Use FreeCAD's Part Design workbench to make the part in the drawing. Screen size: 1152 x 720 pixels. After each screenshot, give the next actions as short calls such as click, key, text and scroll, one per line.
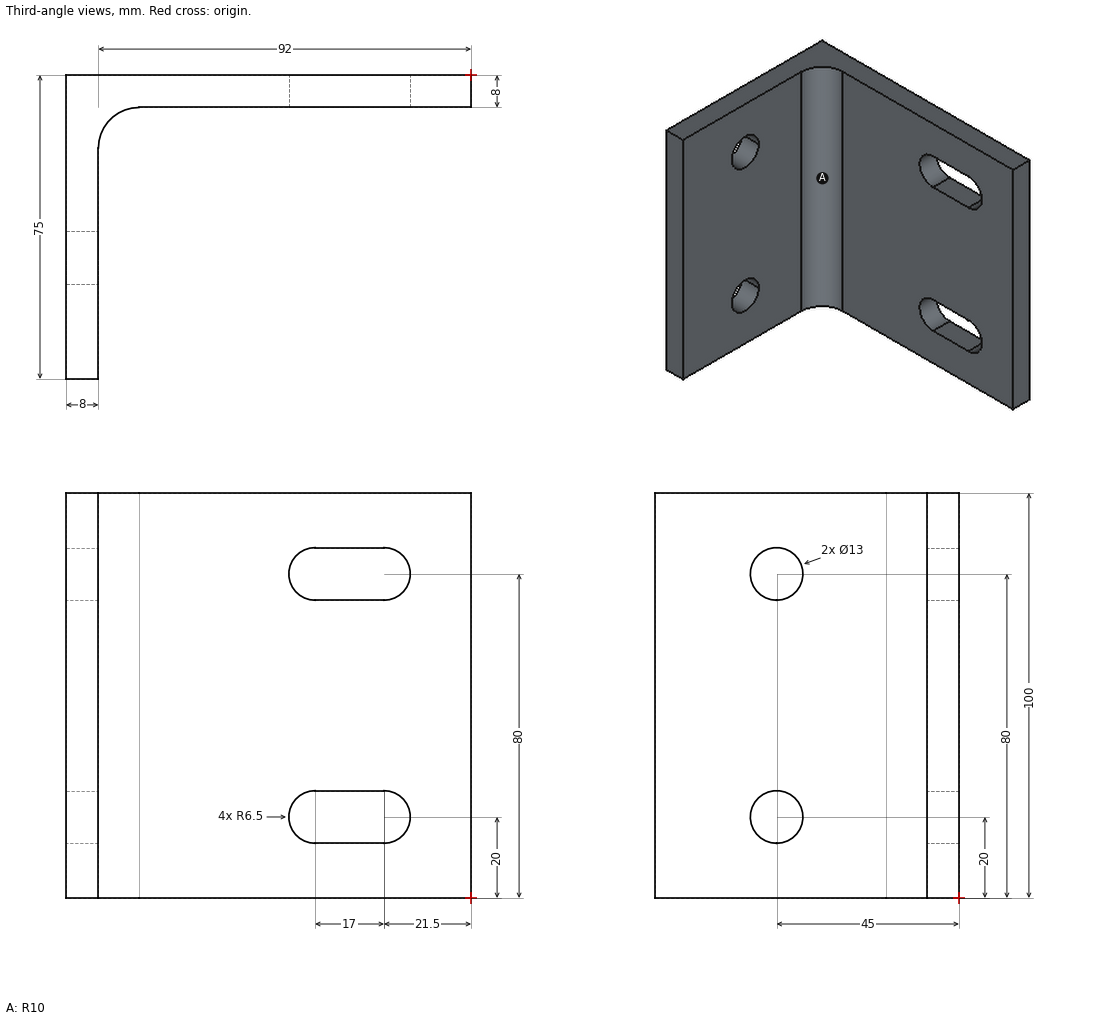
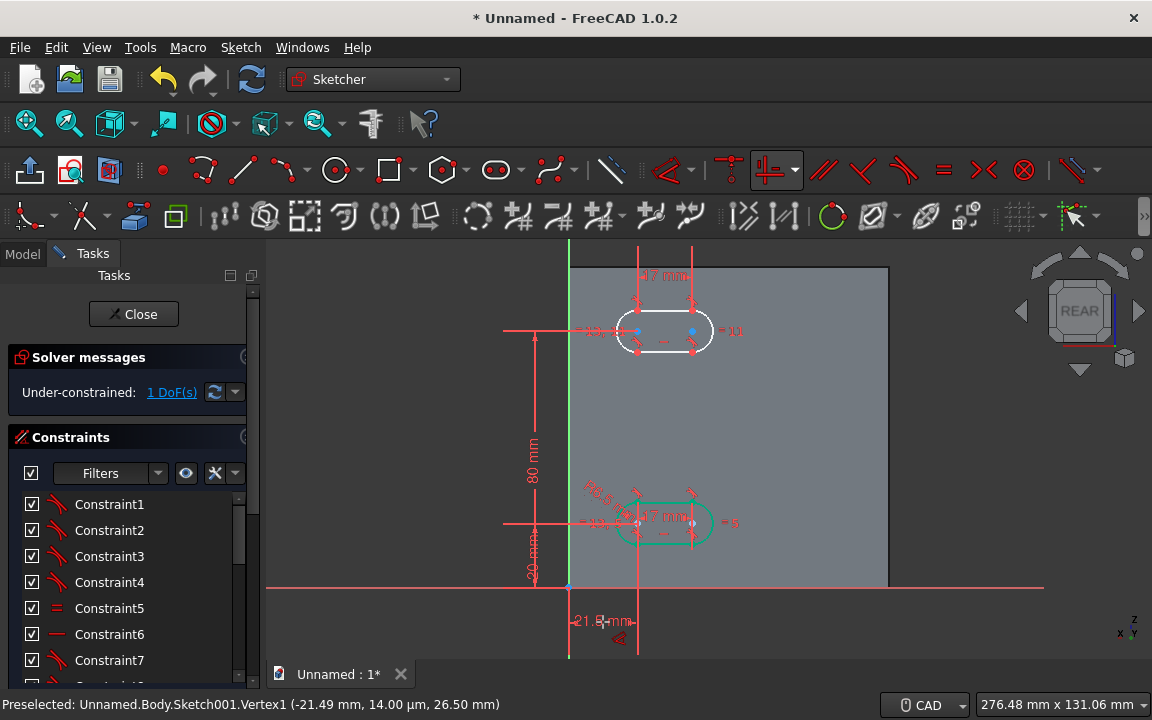
click(638, 311)
click(587, 277)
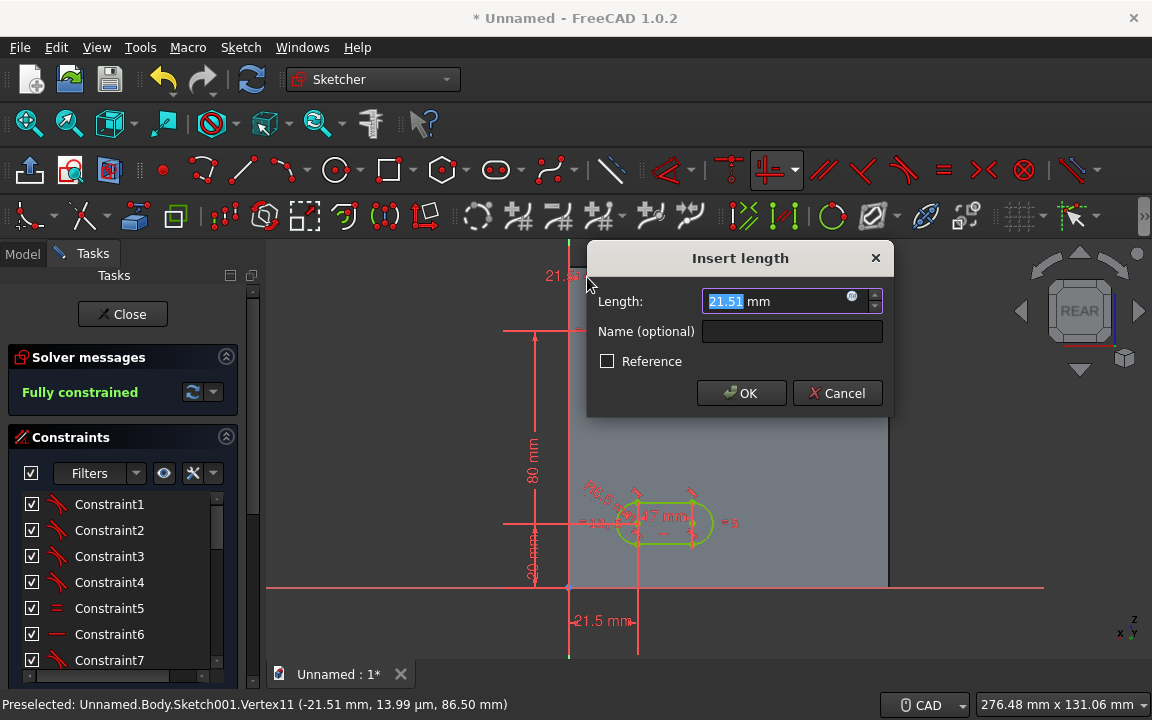
text(21.5)
key(Return)
key(Escape)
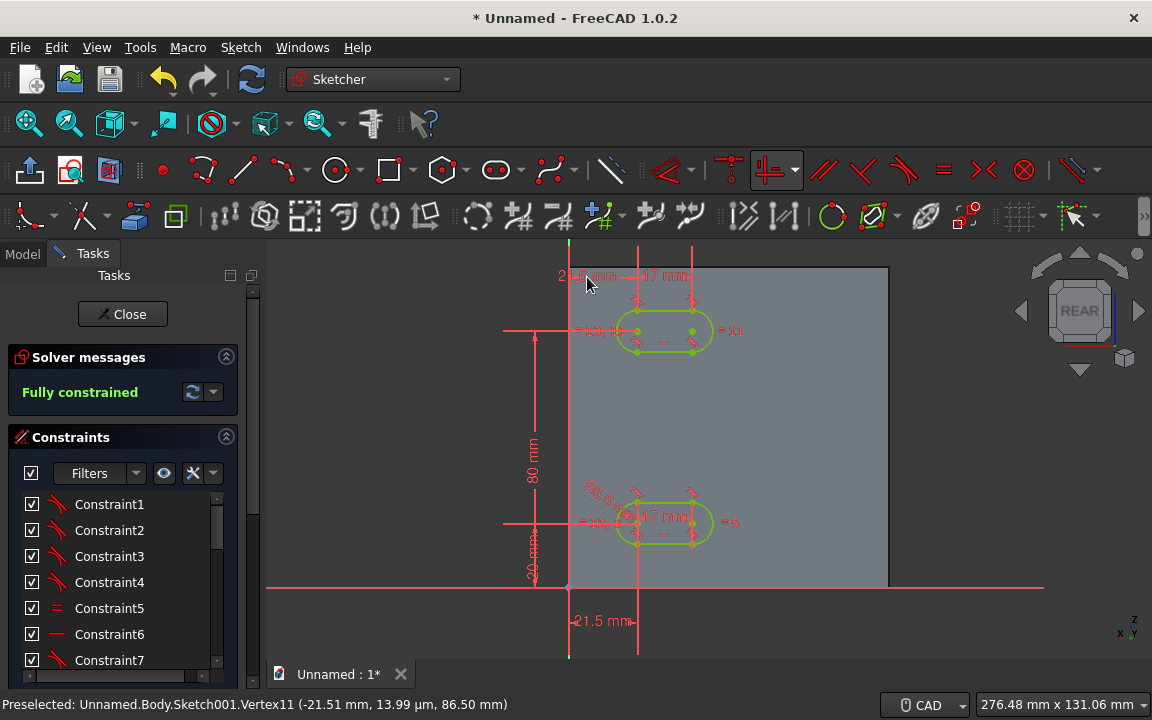
click(123, 314)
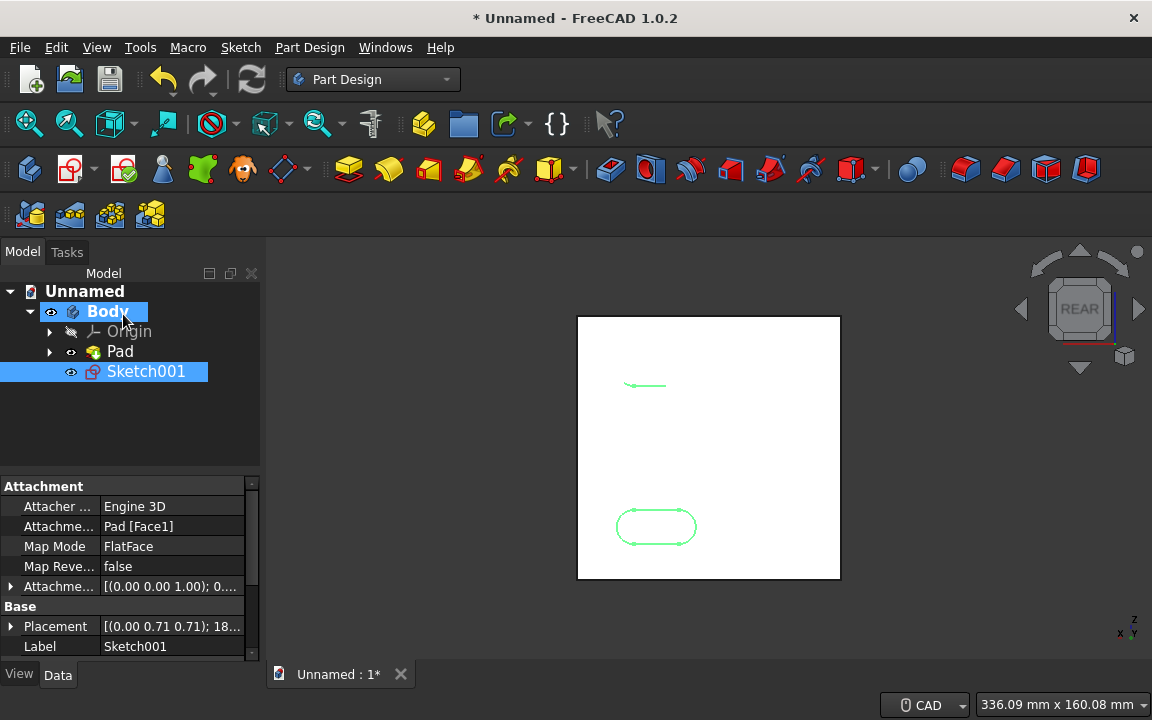
click(612, 170)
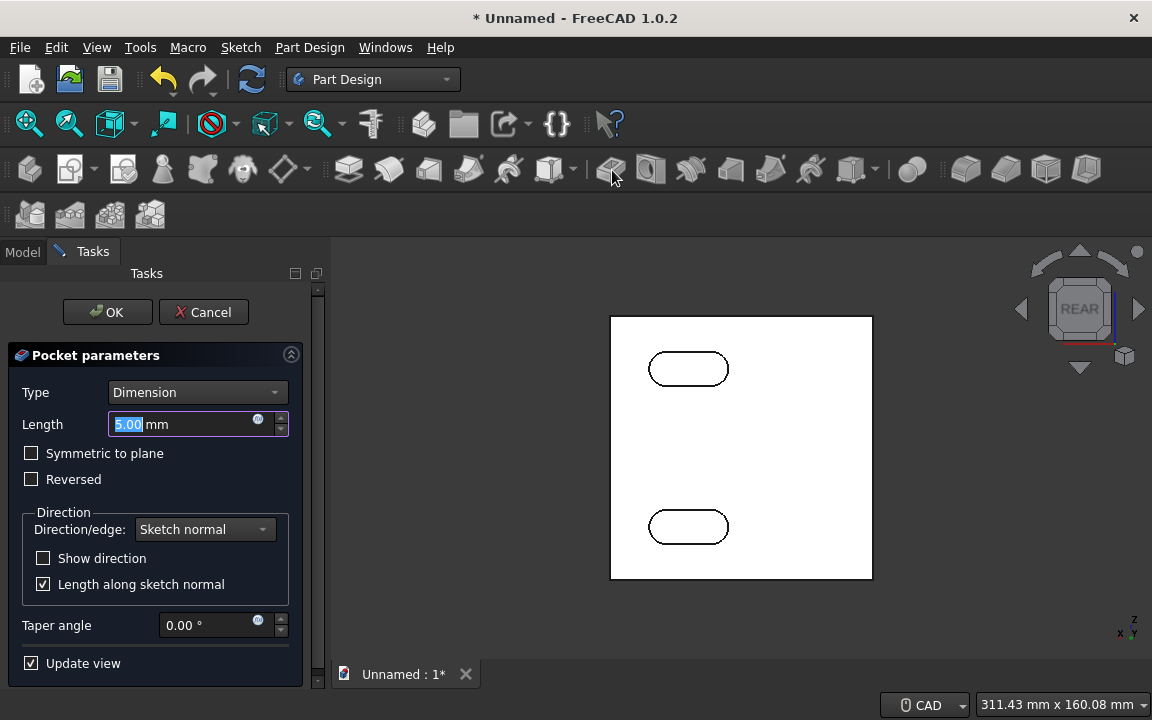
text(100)
key(Tab)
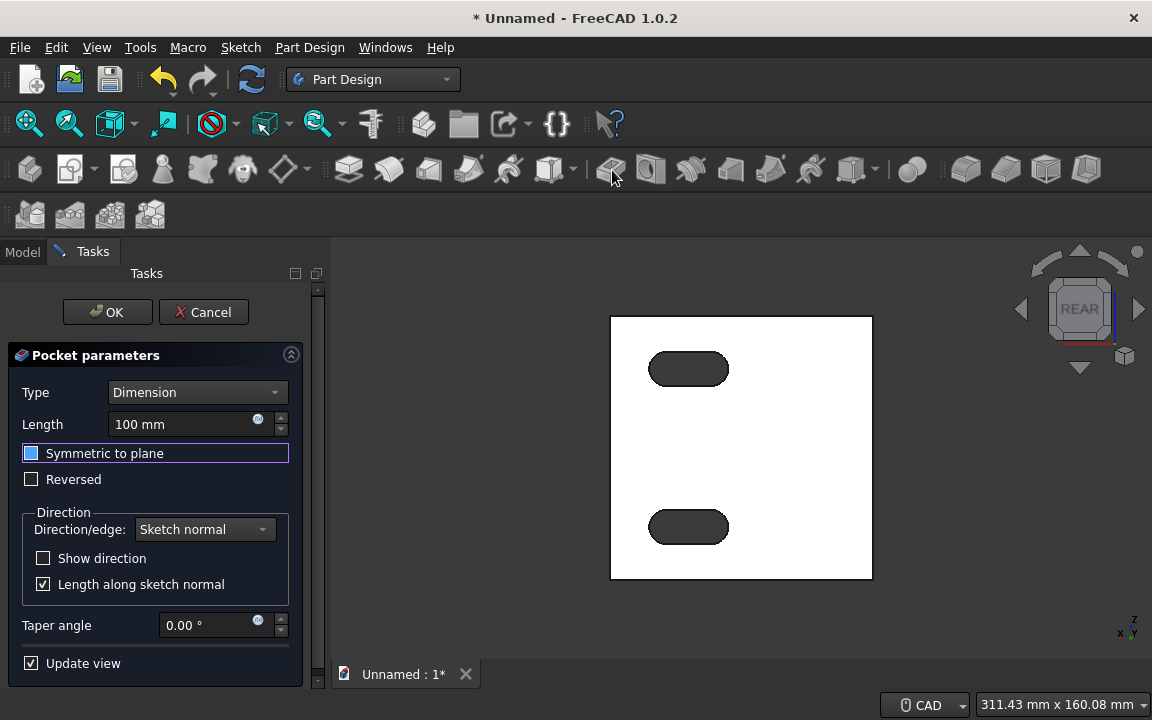
click(108, 312)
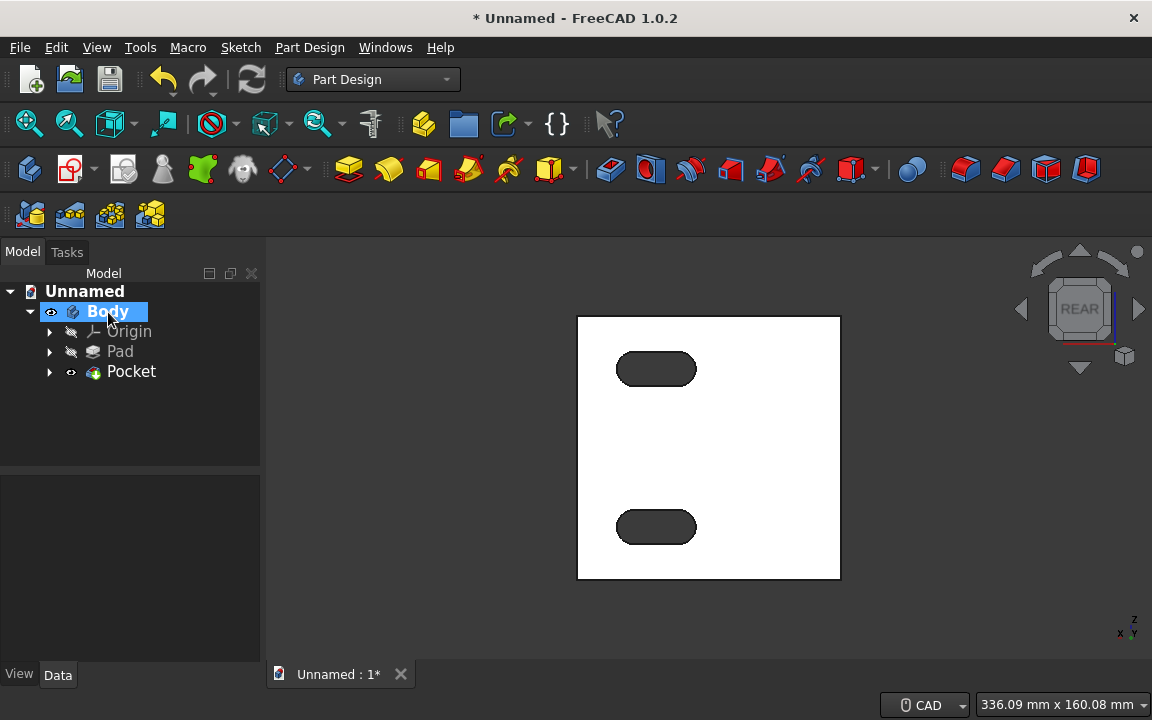
key(0)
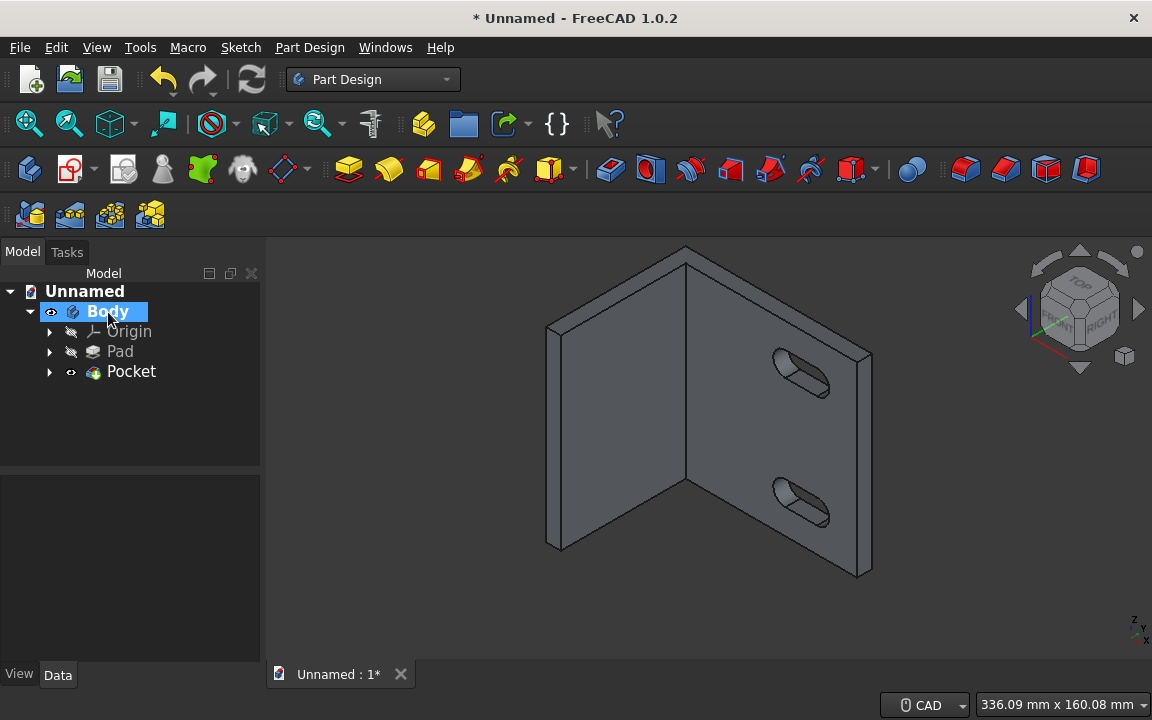
click(623, 375)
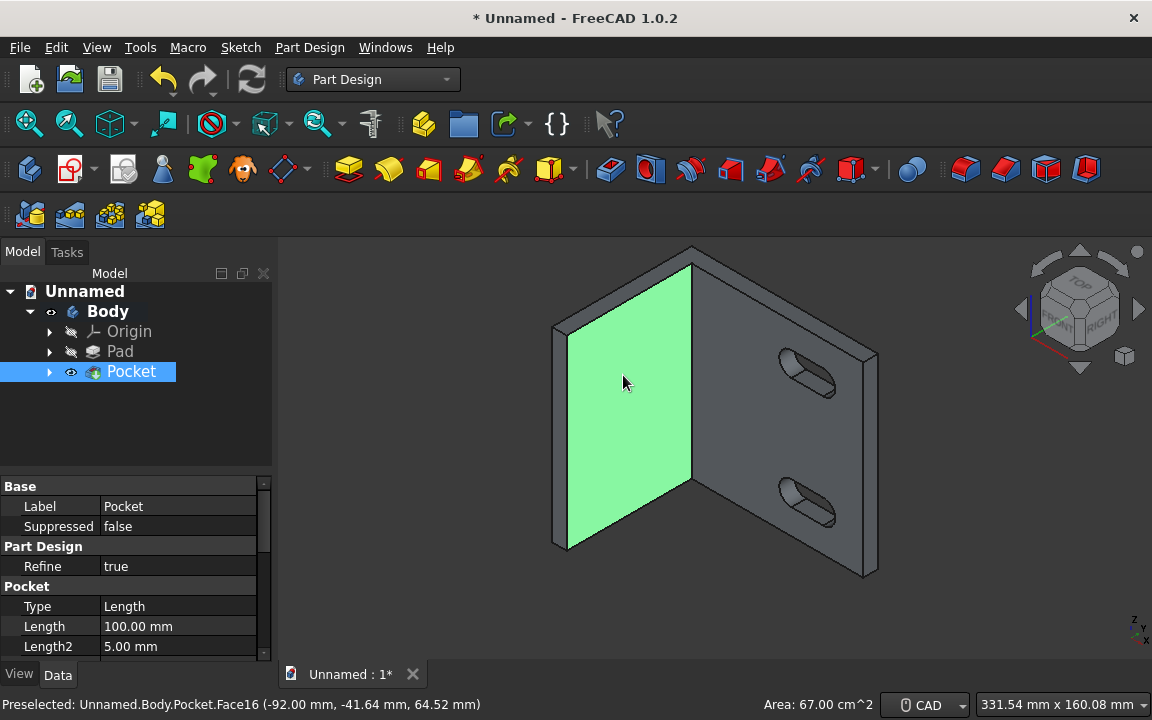
click(70, 170)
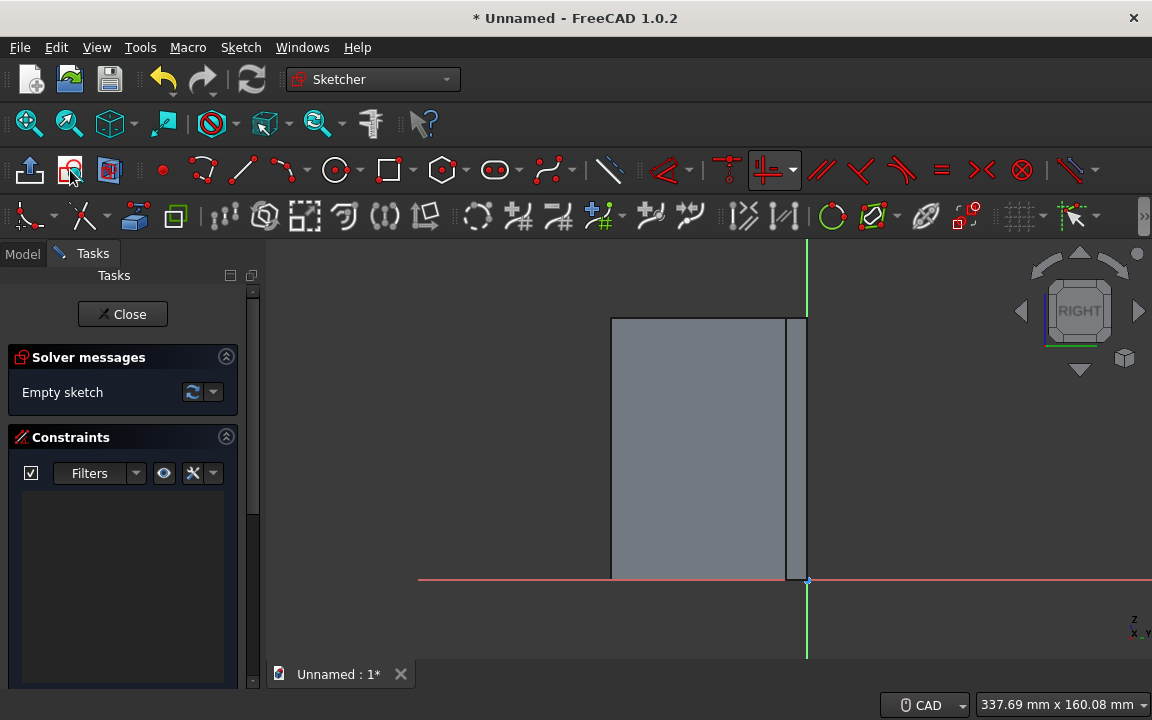
click(336, 170)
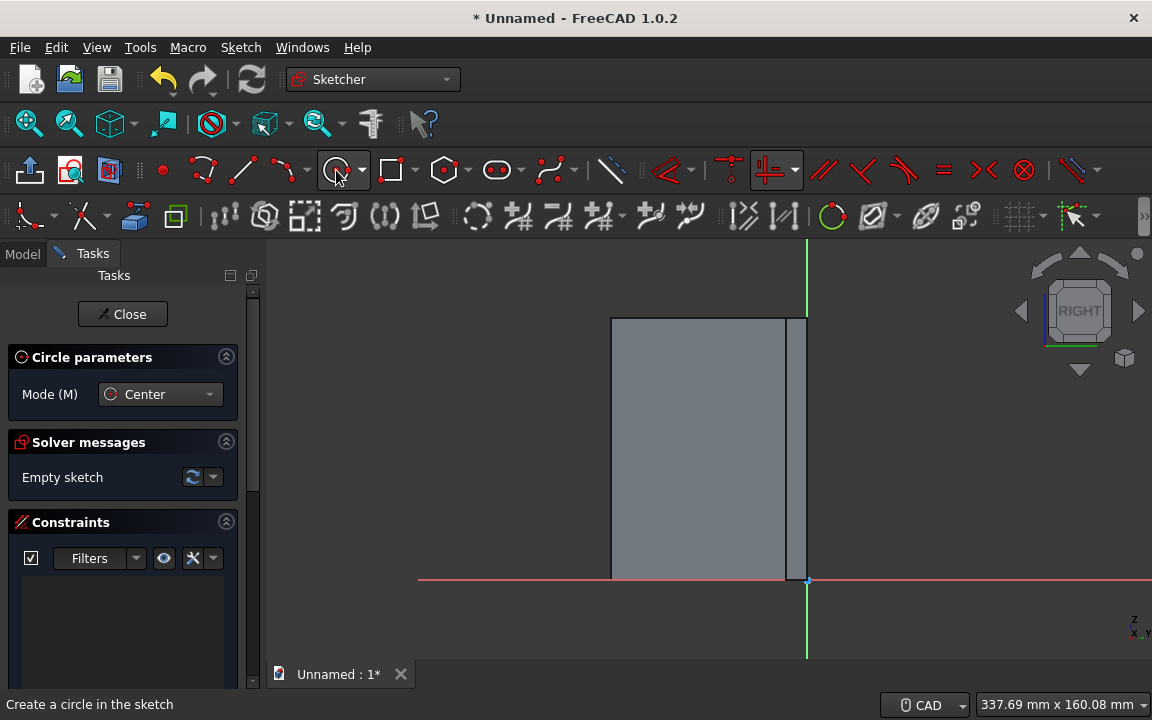
scroll(689, 370, up, 2)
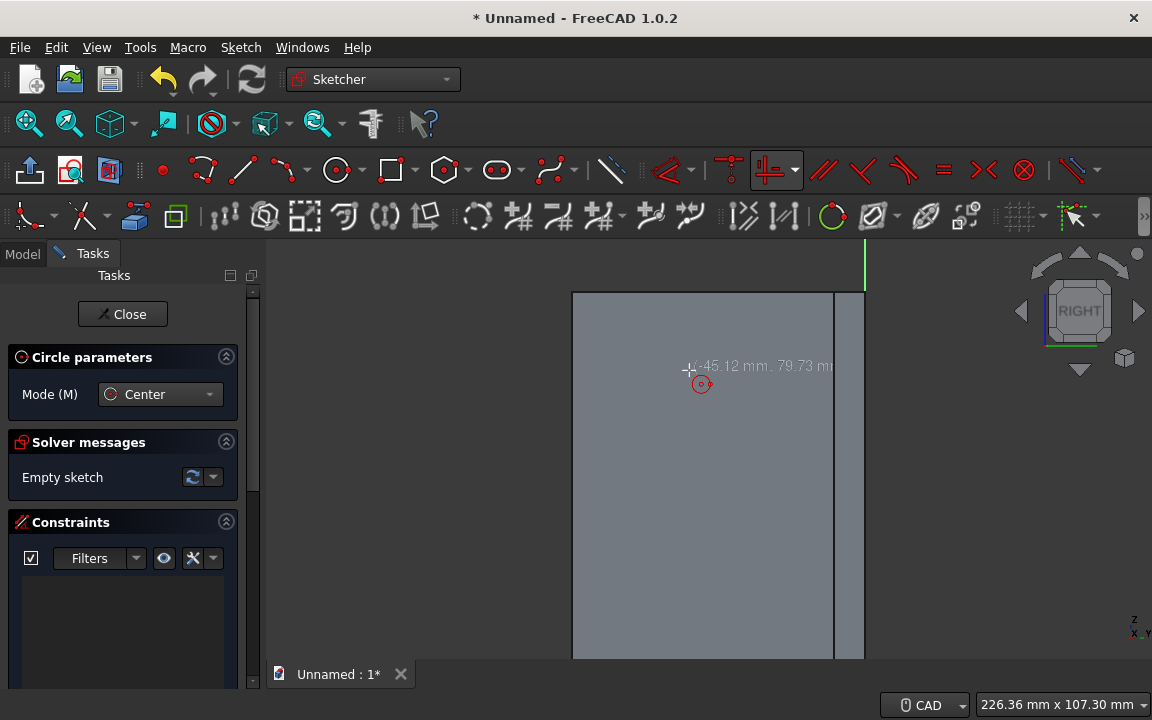
click(689, 370)
move(707, 352)